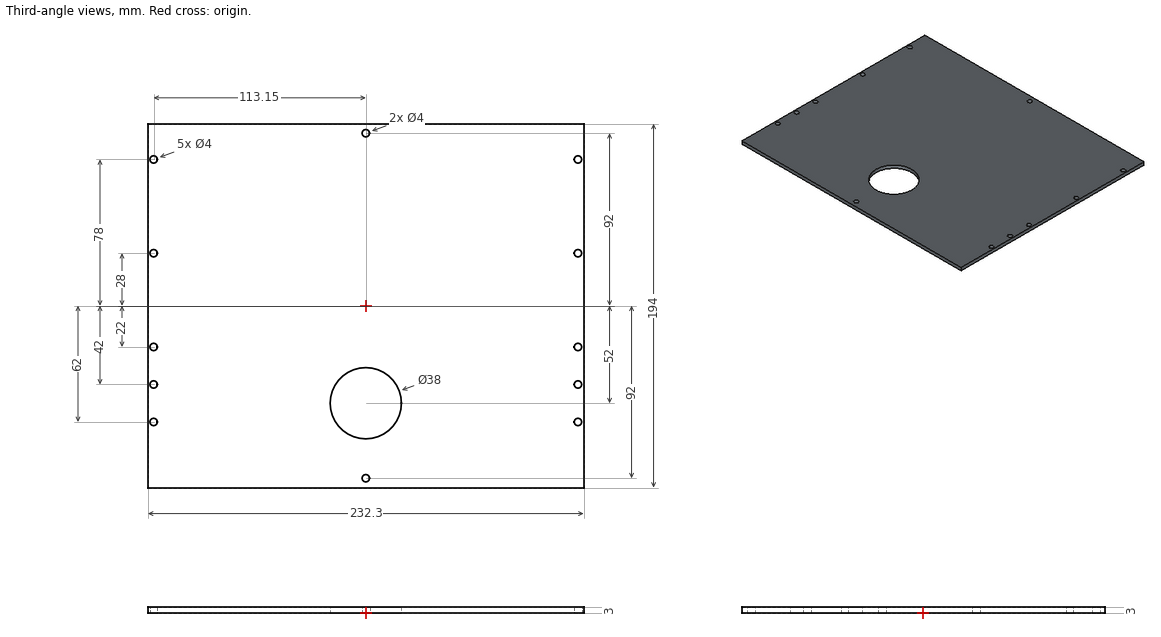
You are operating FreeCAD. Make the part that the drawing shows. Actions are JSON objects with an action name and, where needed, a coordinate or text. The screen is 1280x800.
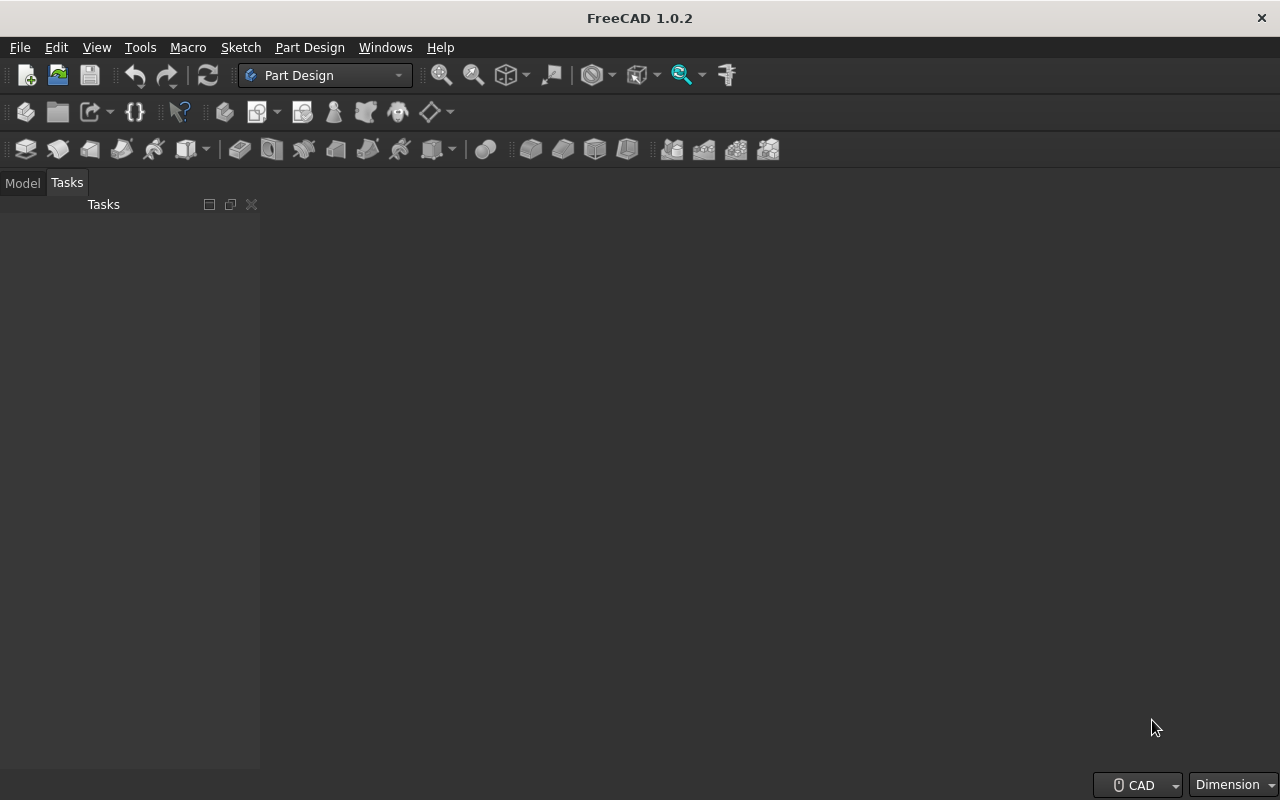
{"action": "key", "text": "ctrl+n"}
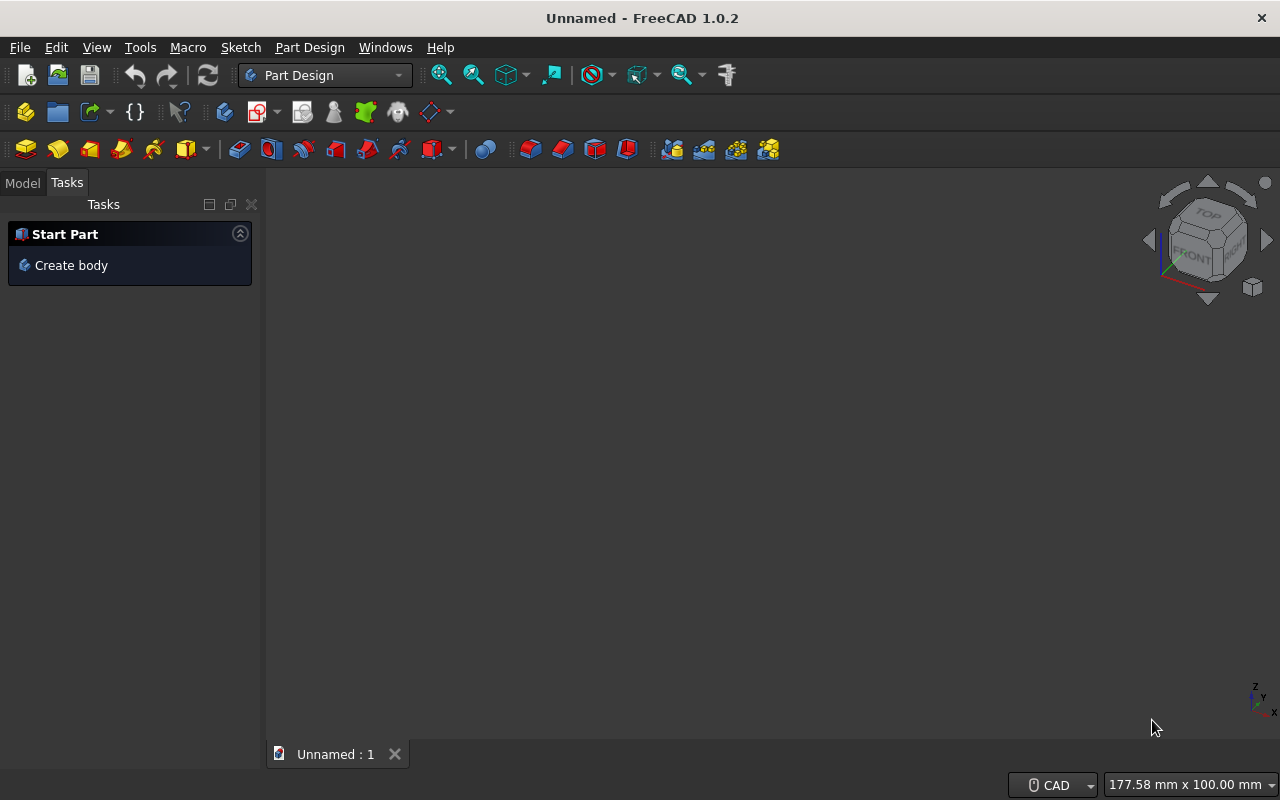
{"action": "left_click", "coordinate": [258, 112]}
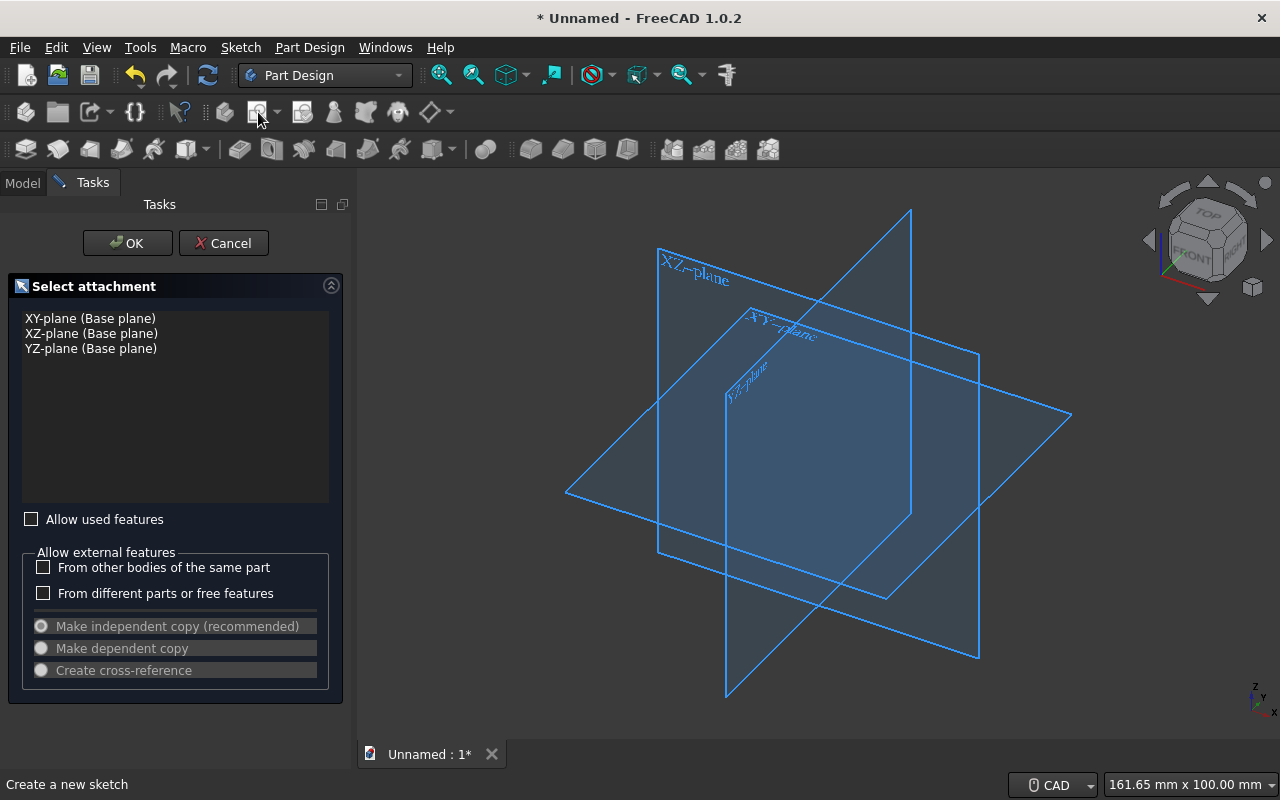
{"action": "left_click", "coordinate": [82, 318]}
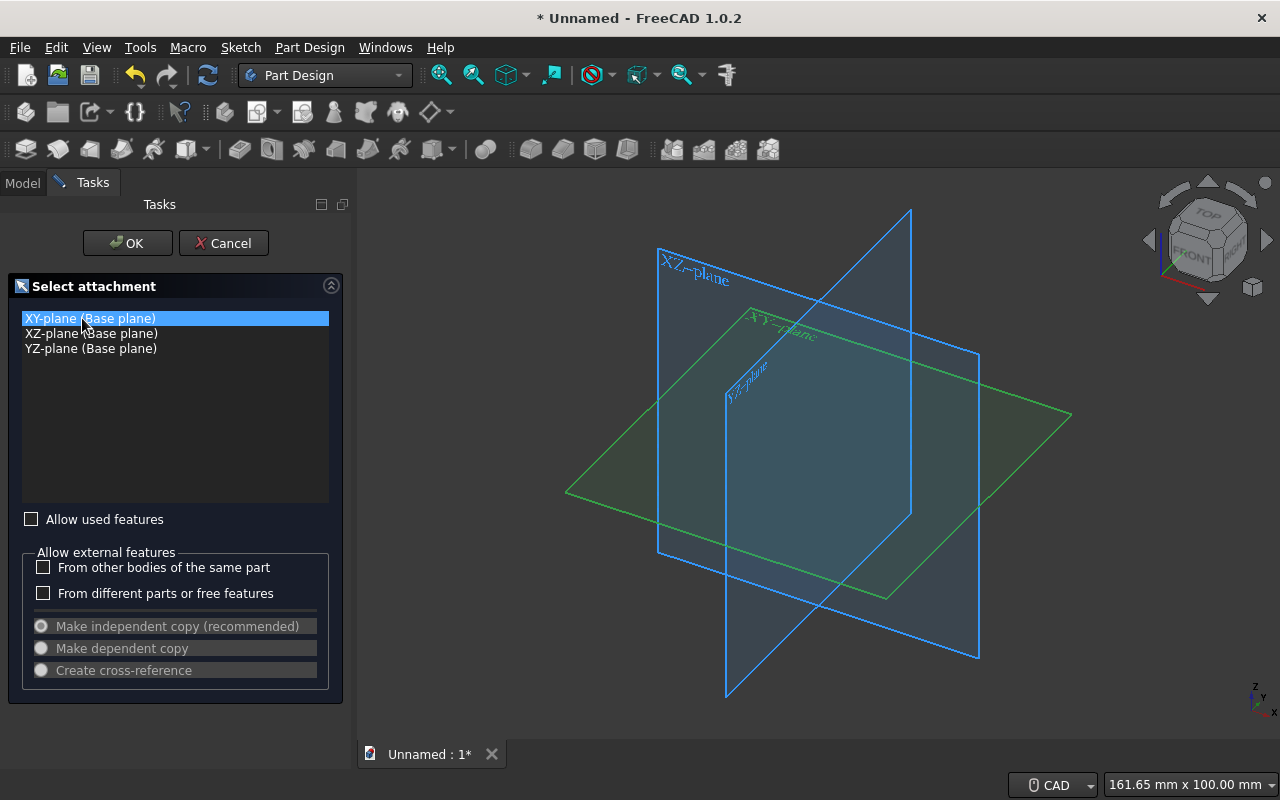
{"action": "left_click", "coordinate": [128, 243]}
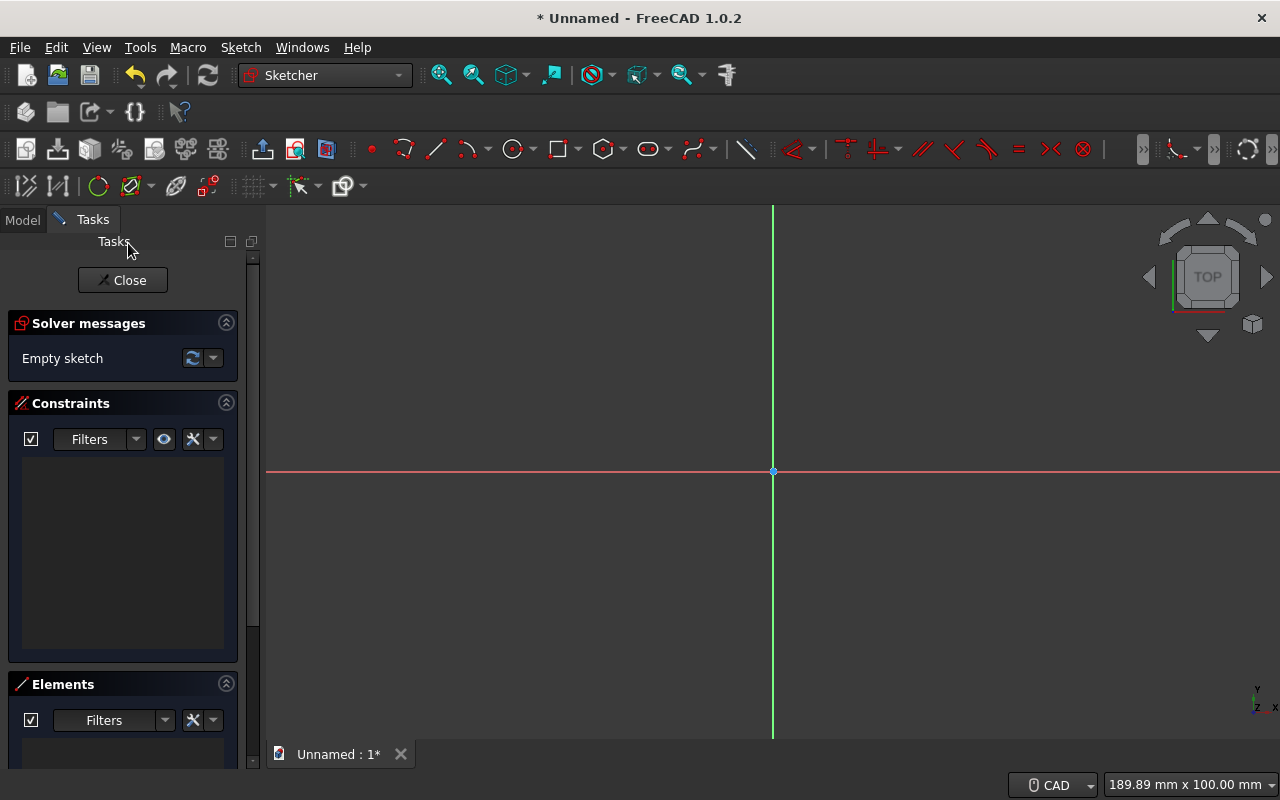
{"action": "scroll", "coordinate": [675, 472], "scroll_direction": "down", "scroll_amount": 6}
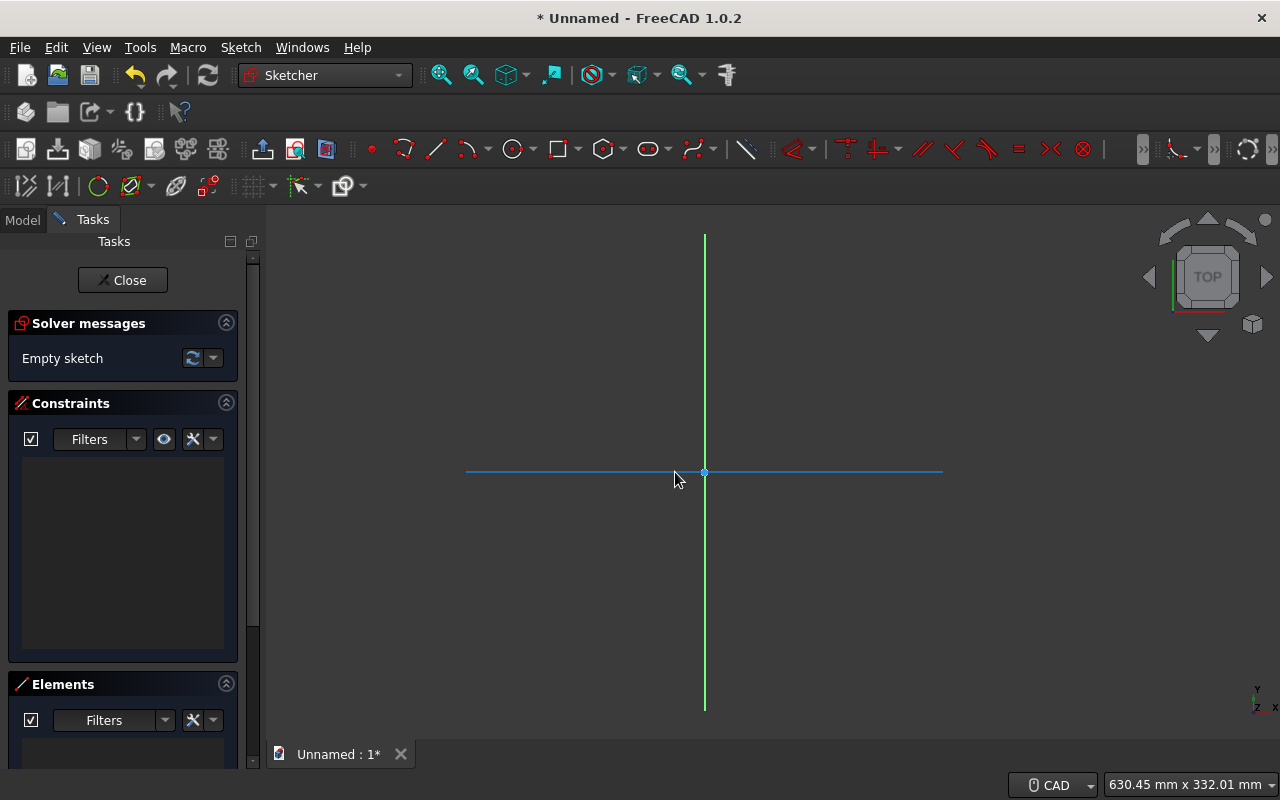
{"action": "key", "text": "g v"}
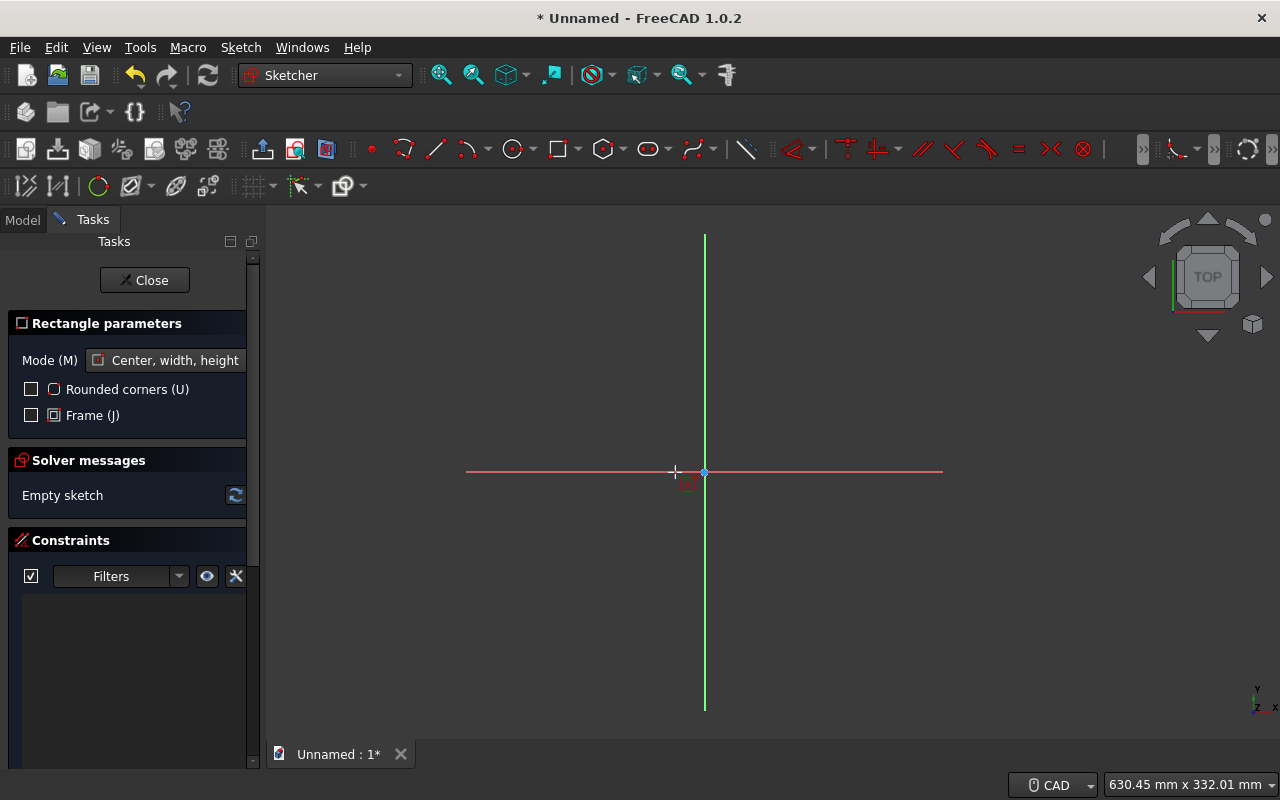
{"action": "left_click", "coordinate": [705, 472]}
{"action": "left_click", "coordinate": [892, 316]}
{"action": "key", "text": "Escape"}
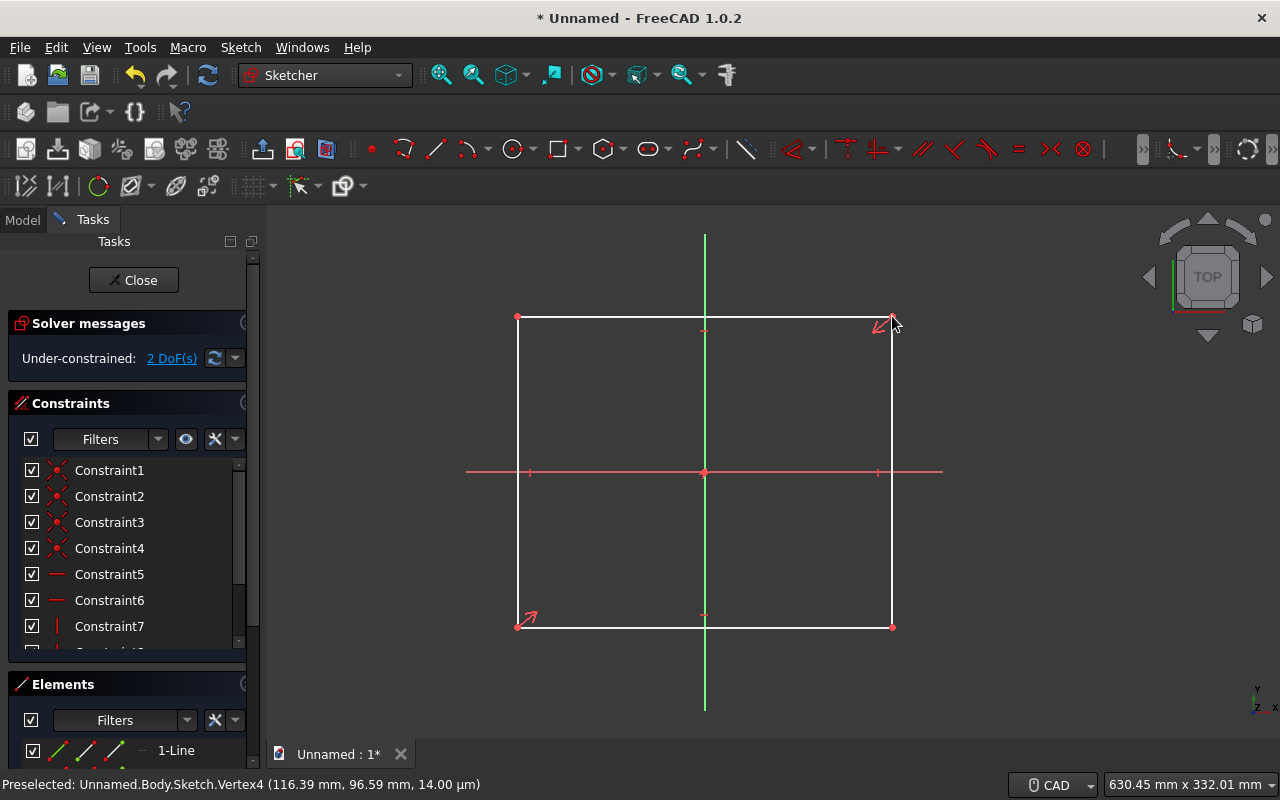
{"action": "left_click", "coordinate": [792, 150]}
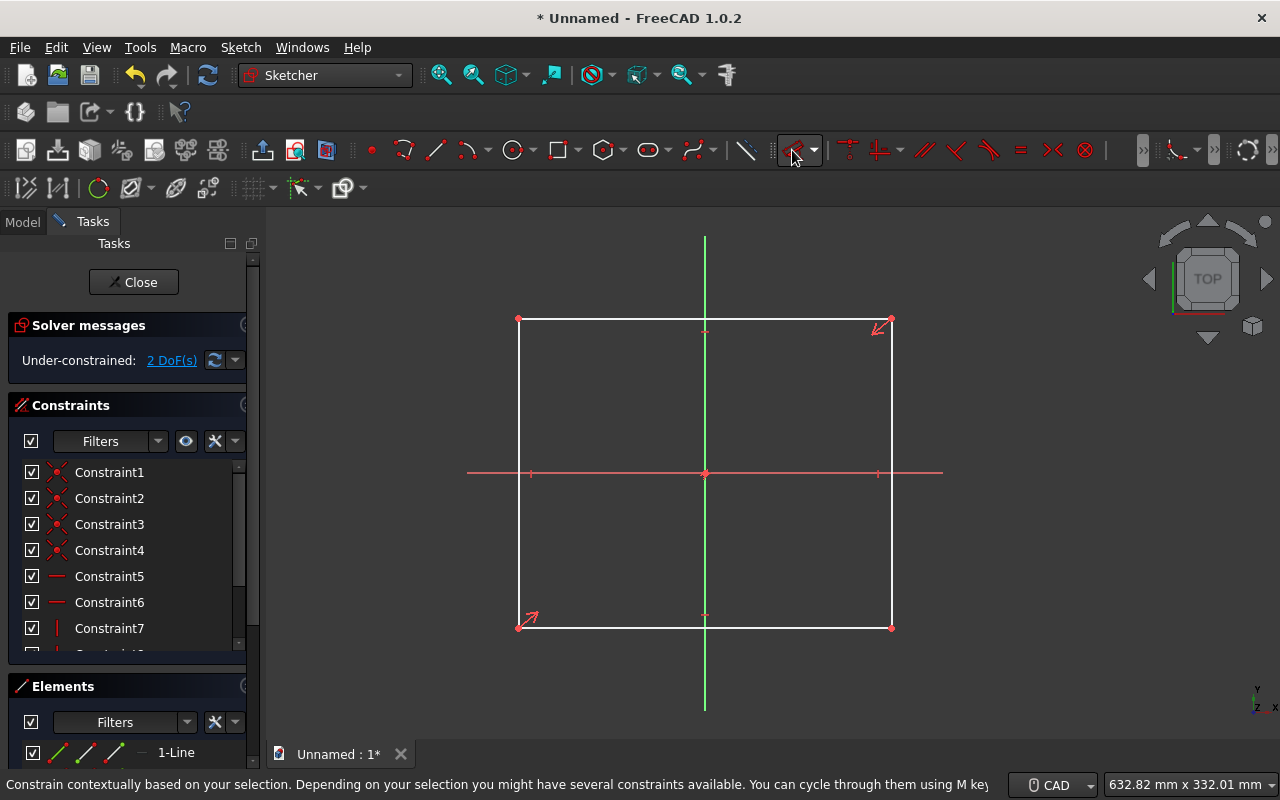
{"action": "left_click", "coordinate": [892, 535]}
{"action": "left_click", "coordinate": [926, 402]}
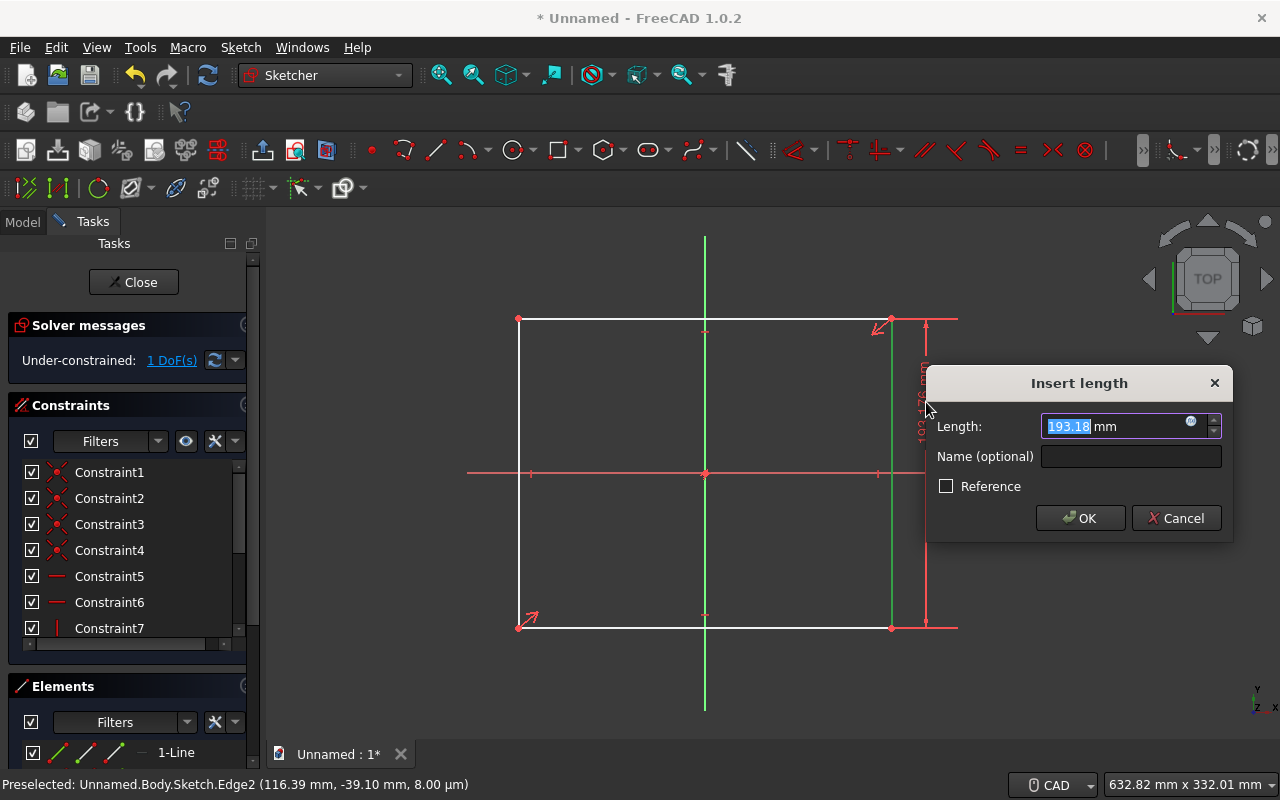
{"action": "type", "text": "194"}
{"action": "key", "text": "Return"}